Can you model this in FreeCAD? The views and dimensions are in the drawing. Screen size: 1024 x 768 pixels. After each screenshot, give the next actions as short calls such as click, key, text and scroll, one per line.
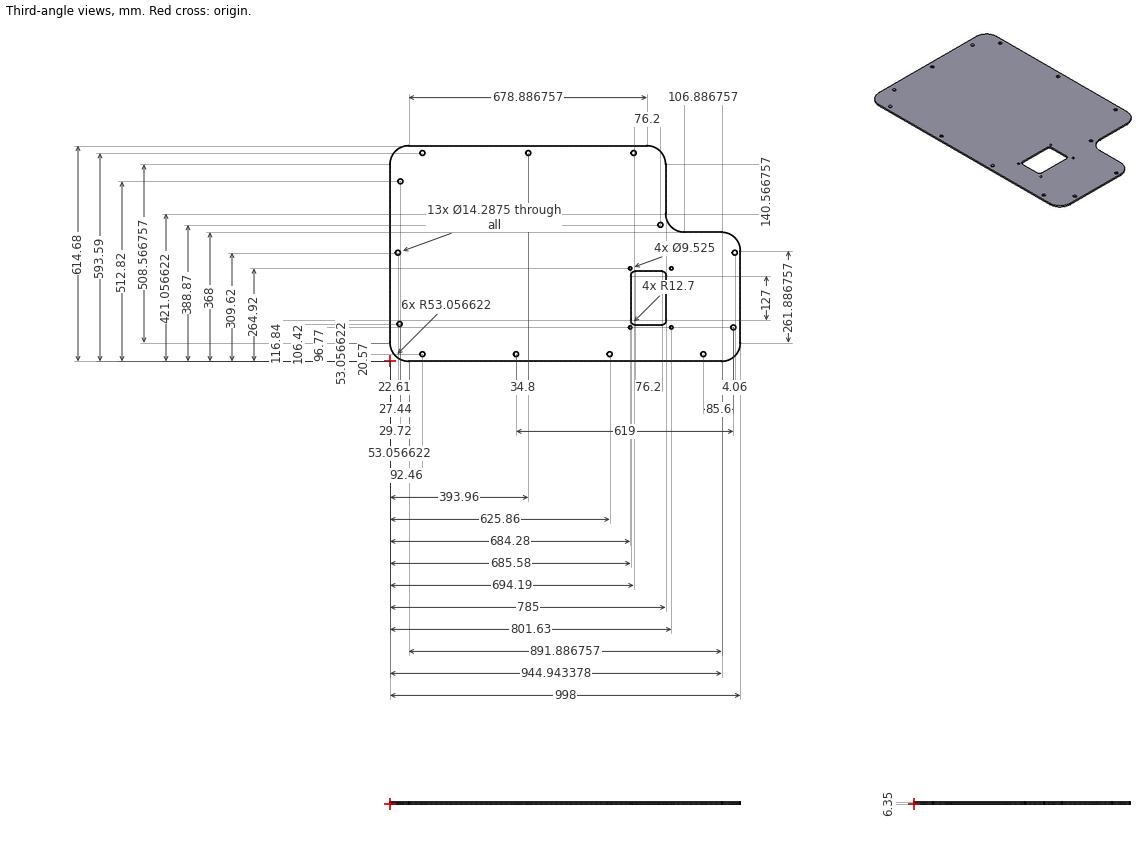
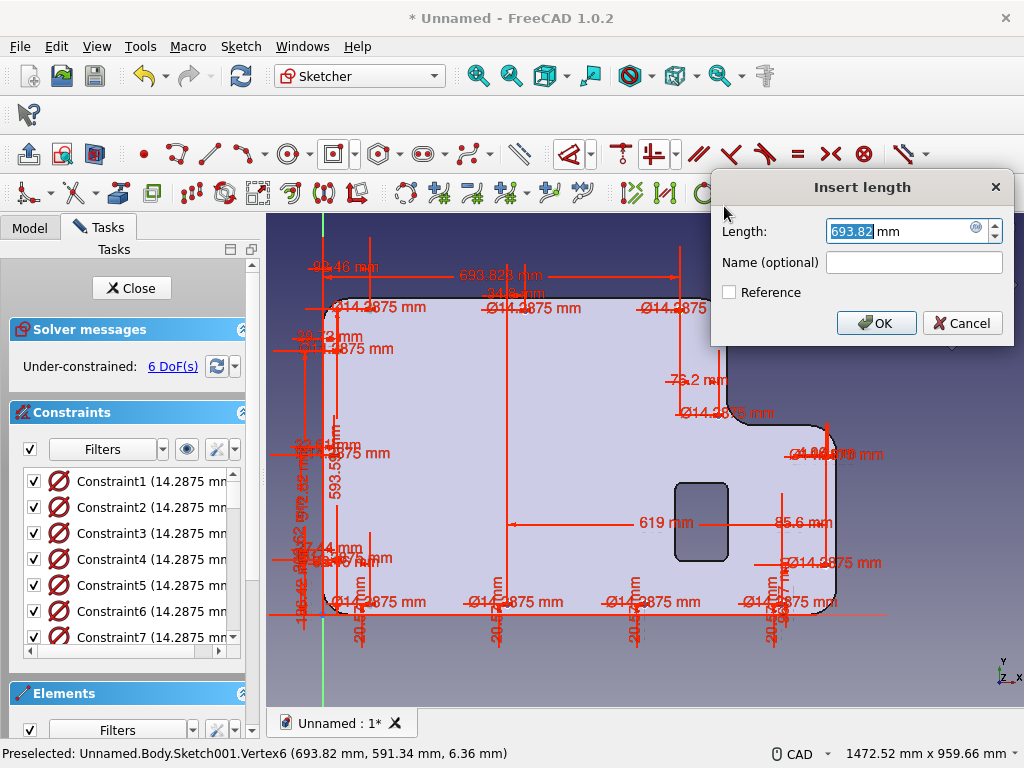
text(694.19)
key(Return)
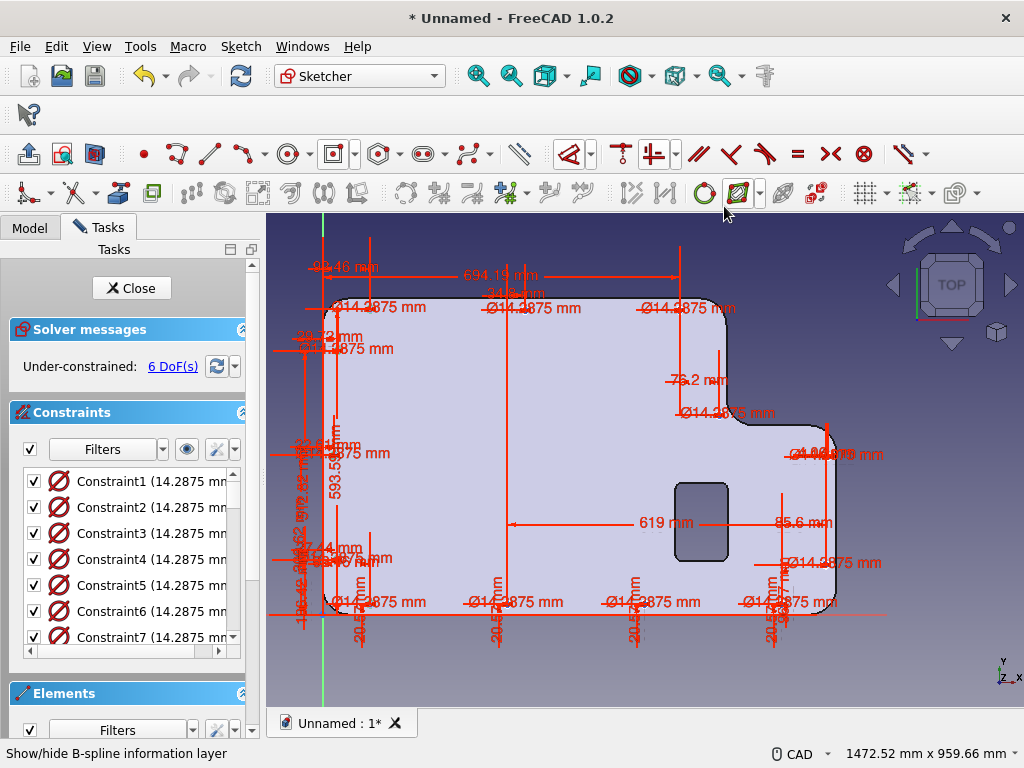
click(680, 310)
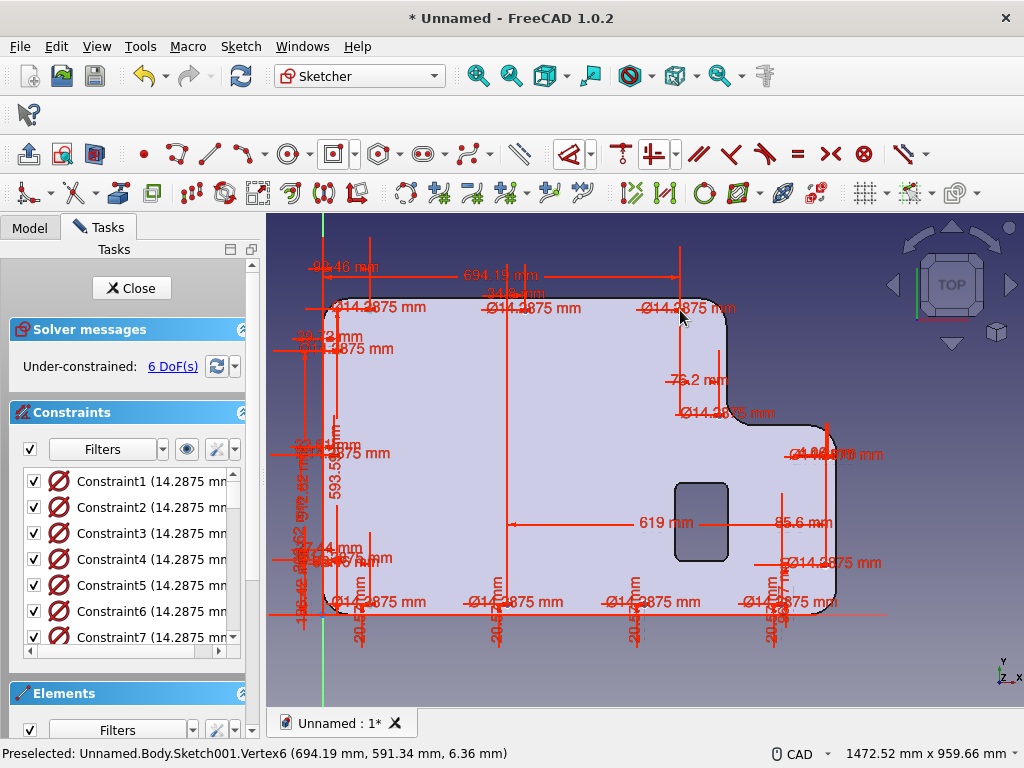
key(i)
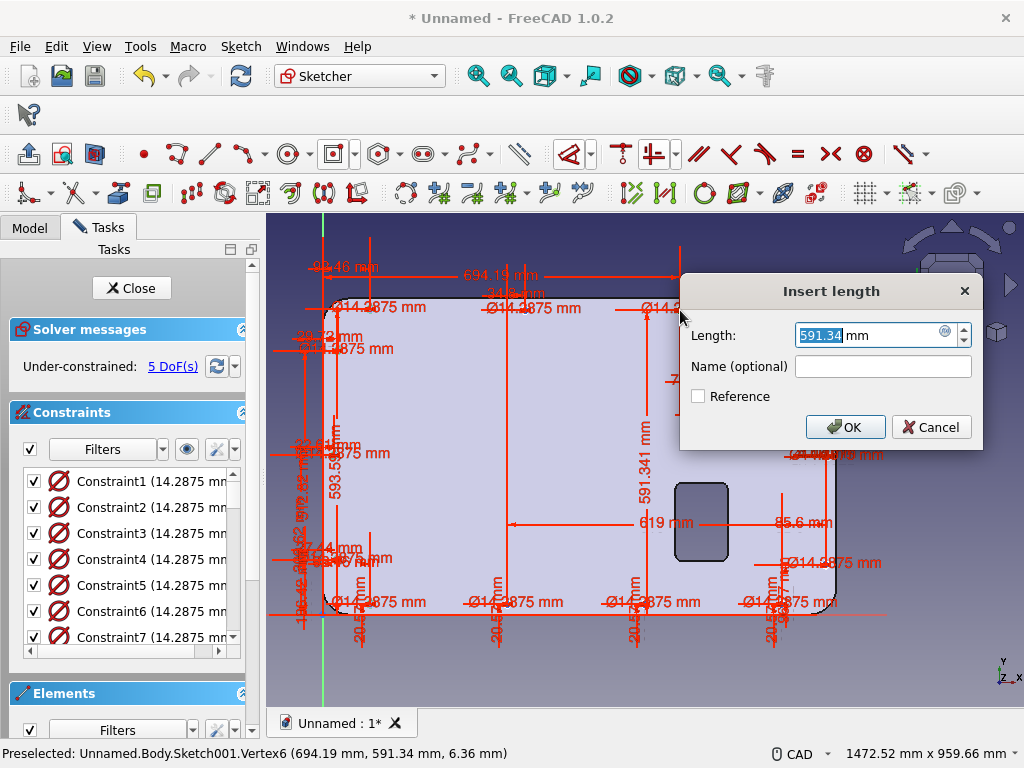
text(593.59)
key(Return)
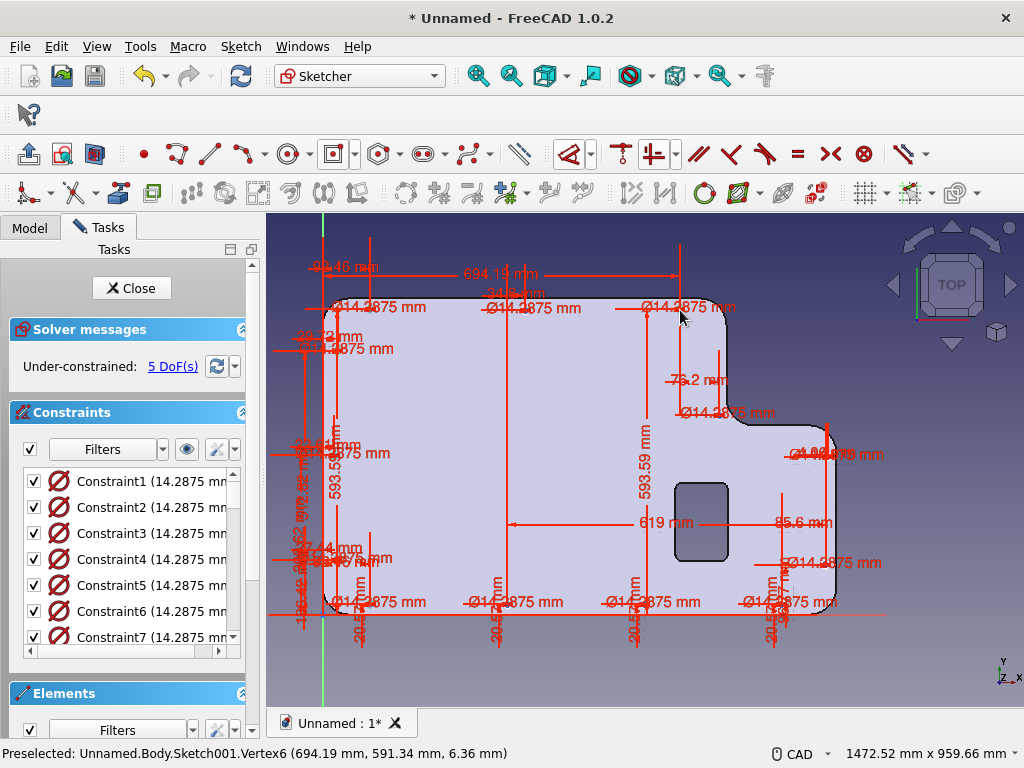
click(525, 310)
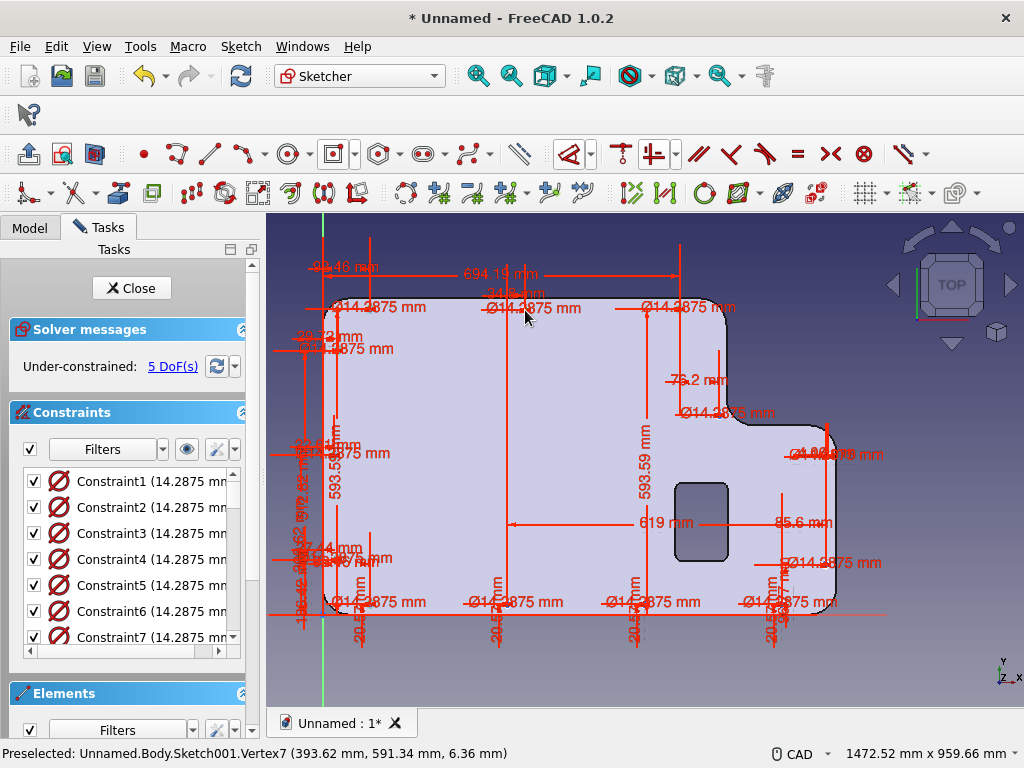
click(590, 154)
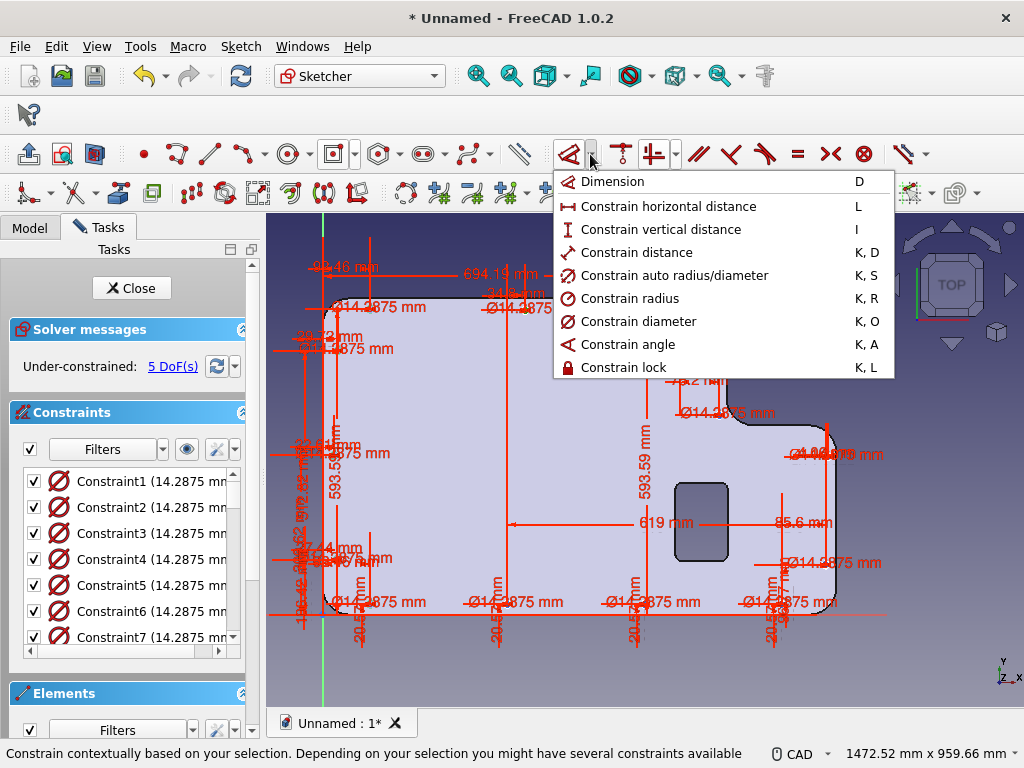
click(724, 206)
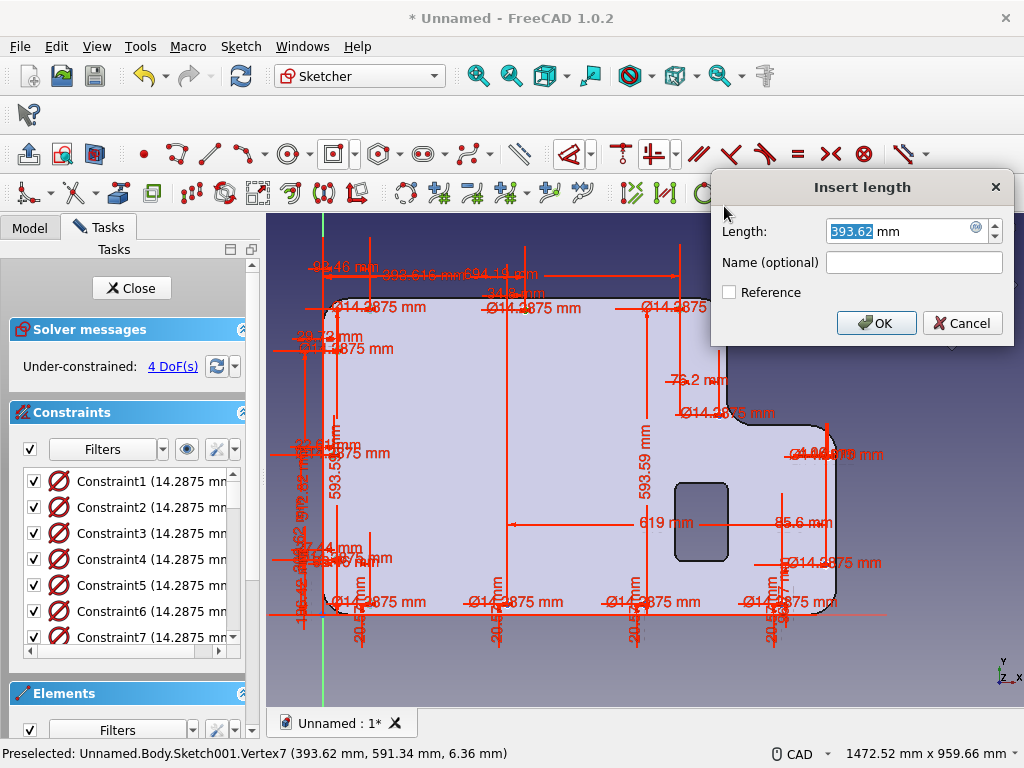
text(393.96)
key(Return)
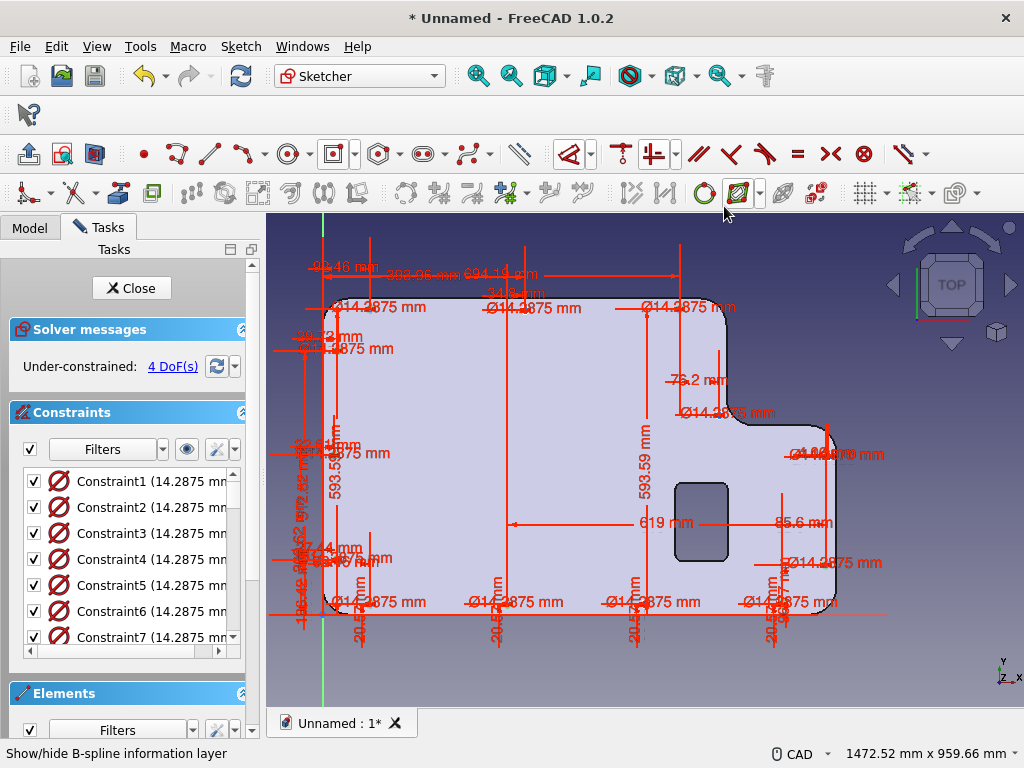
click(525, 310)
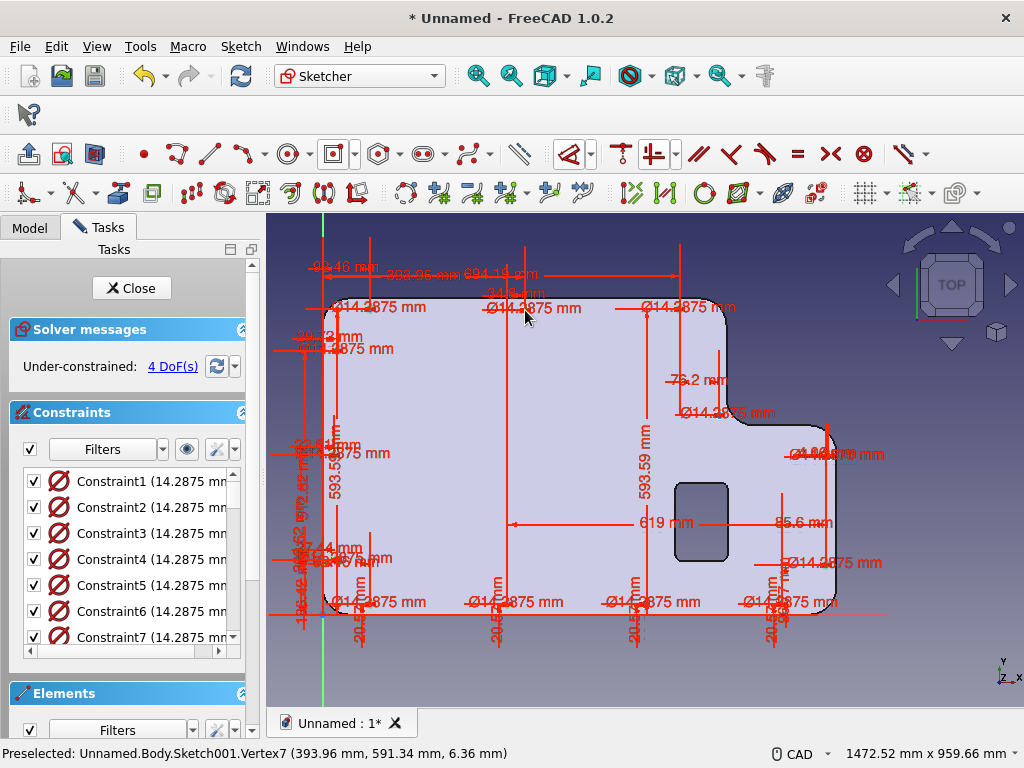
key(i)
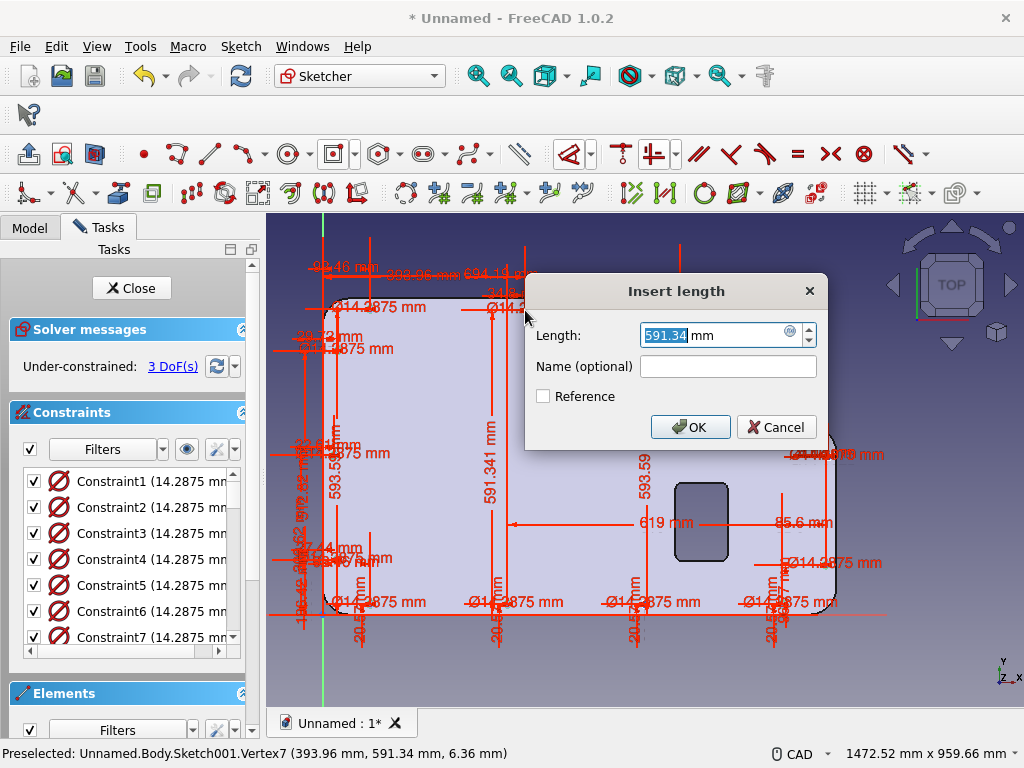
text(593.59)
key(Return)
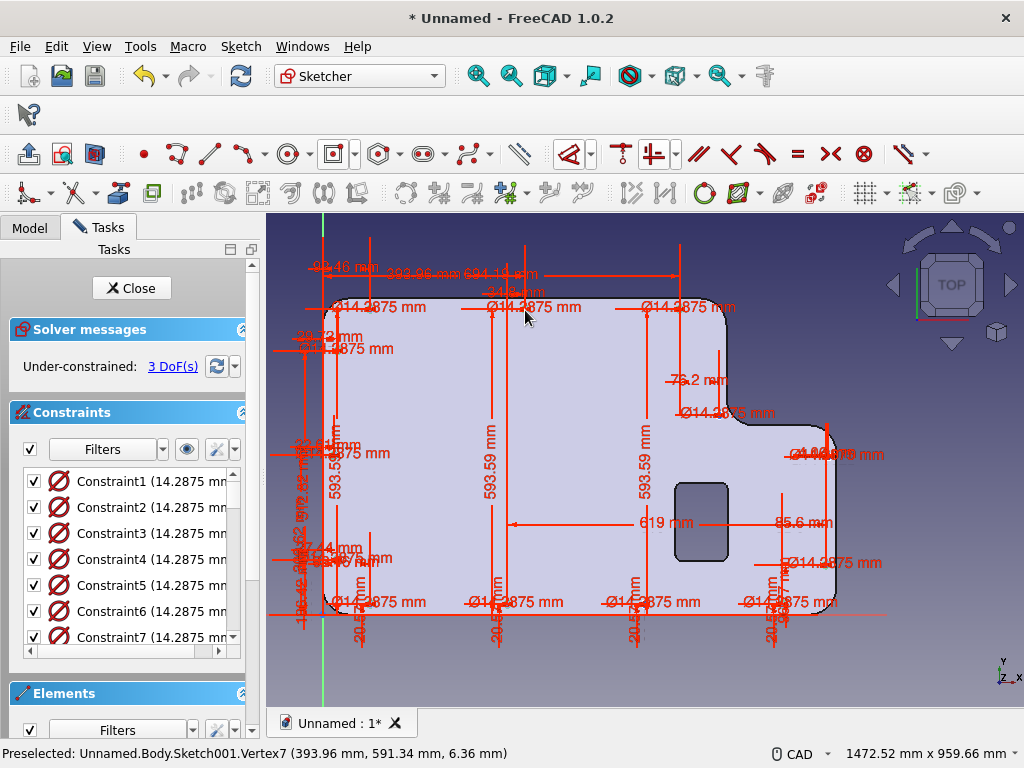
click(645, 604)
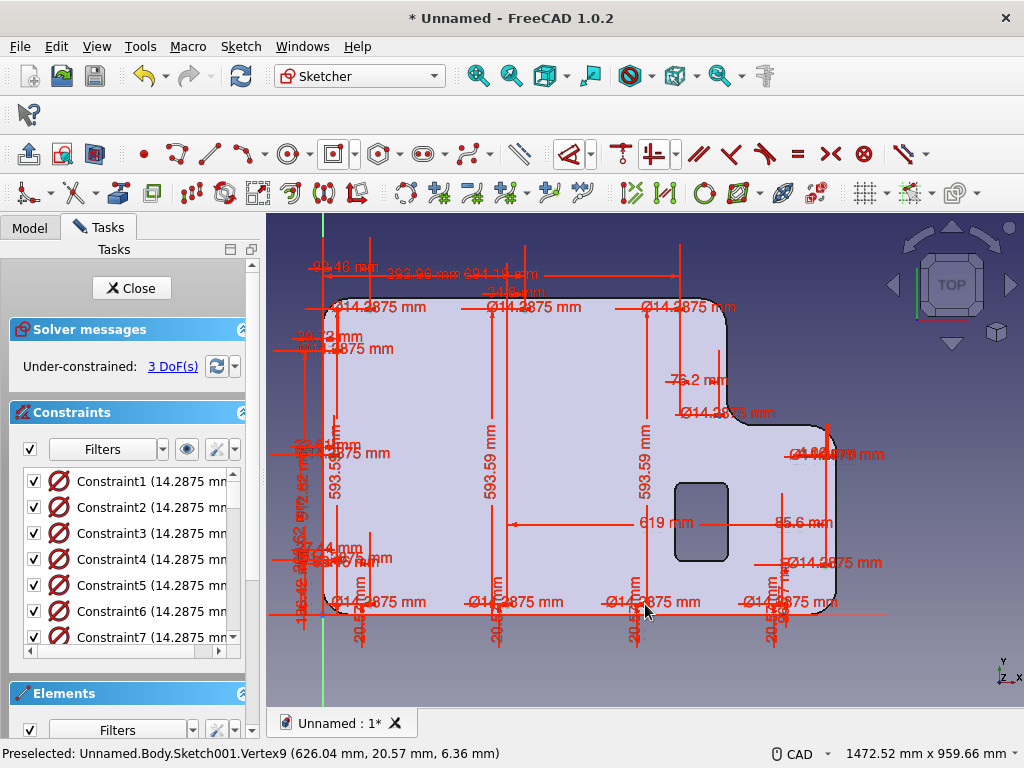
click(590, 154)